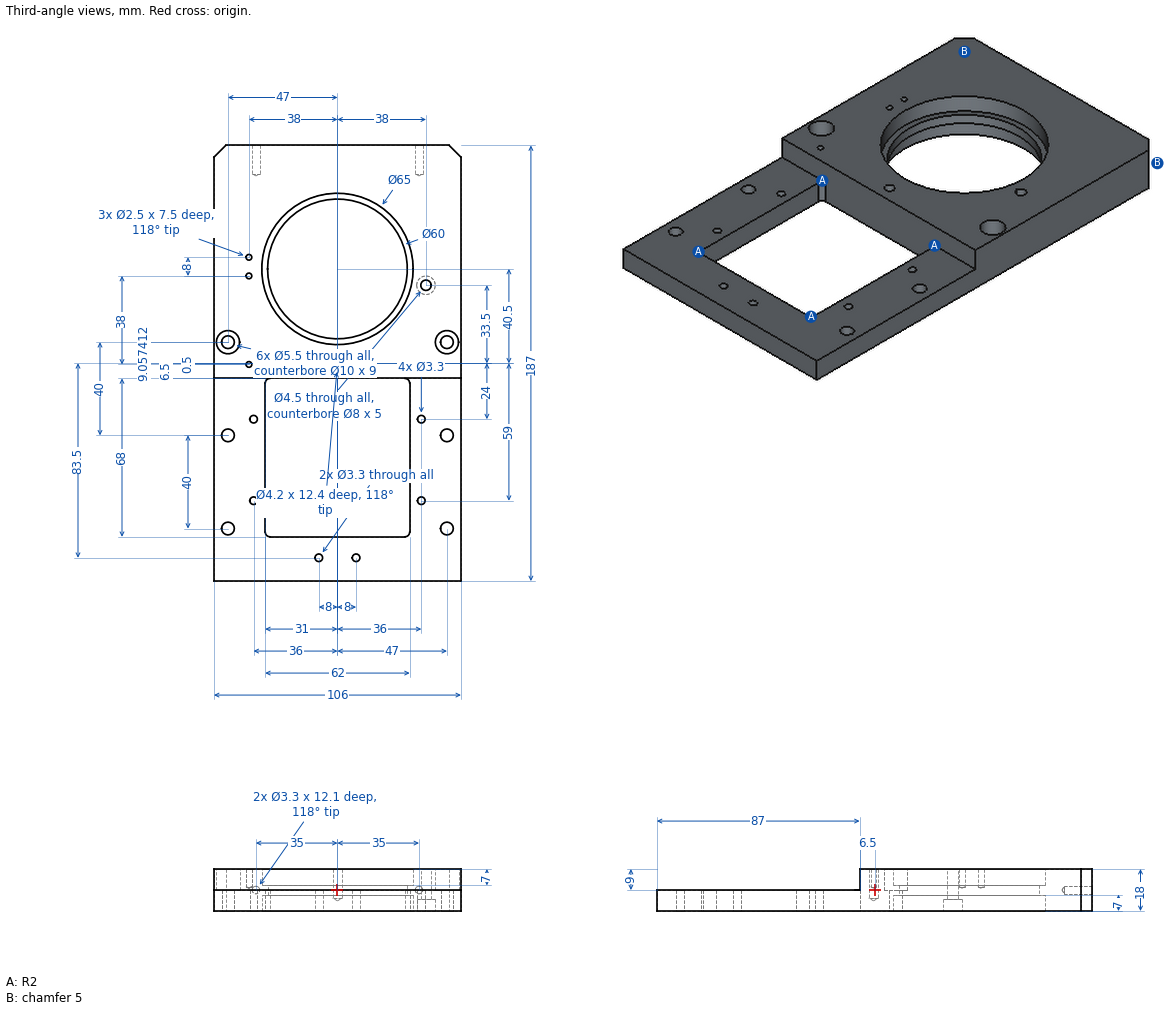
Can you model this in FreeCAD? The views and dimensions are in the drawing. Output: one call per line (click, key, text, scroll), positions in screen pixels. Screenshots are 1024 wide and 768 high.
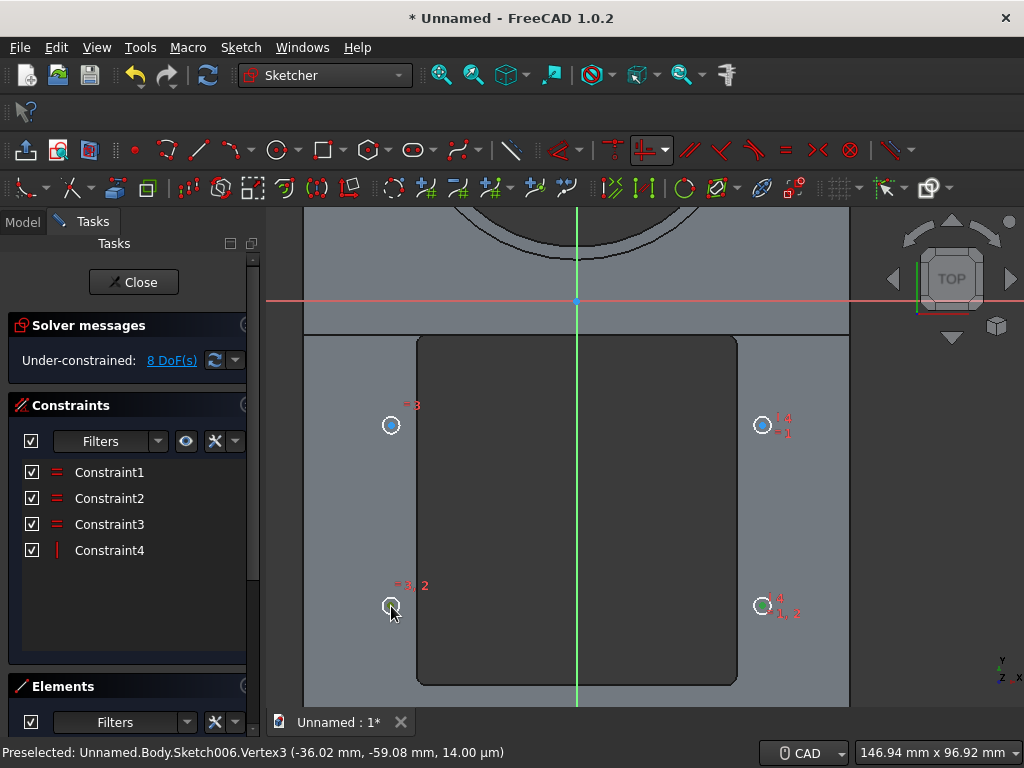
key(h)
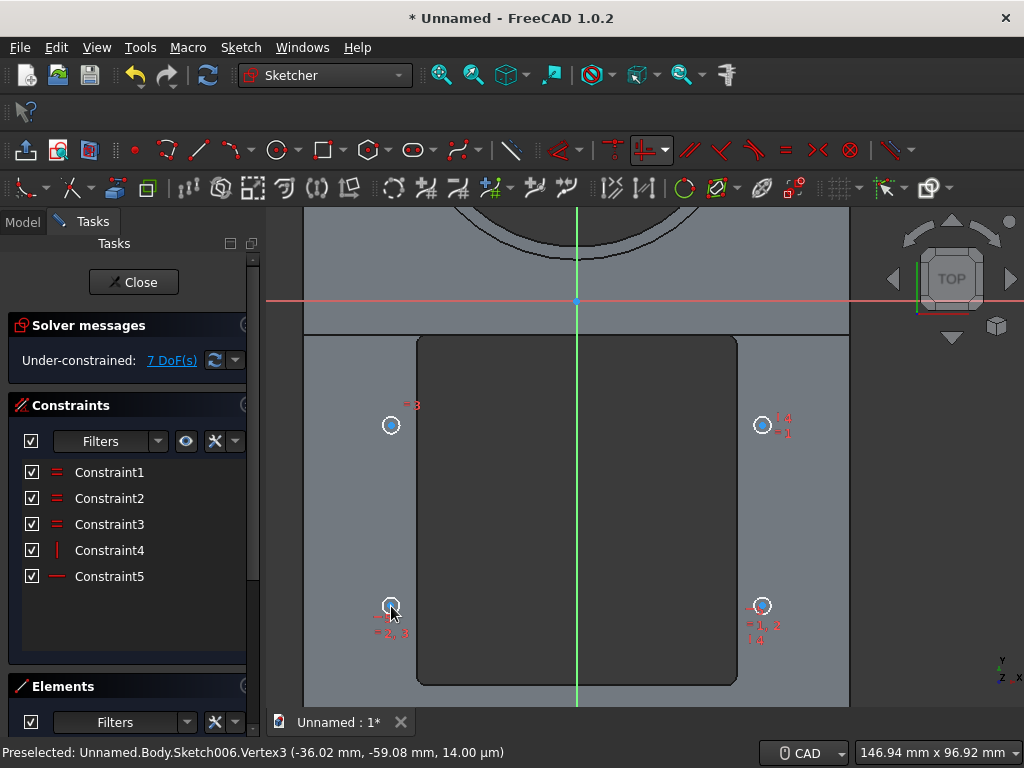
click(391, 606)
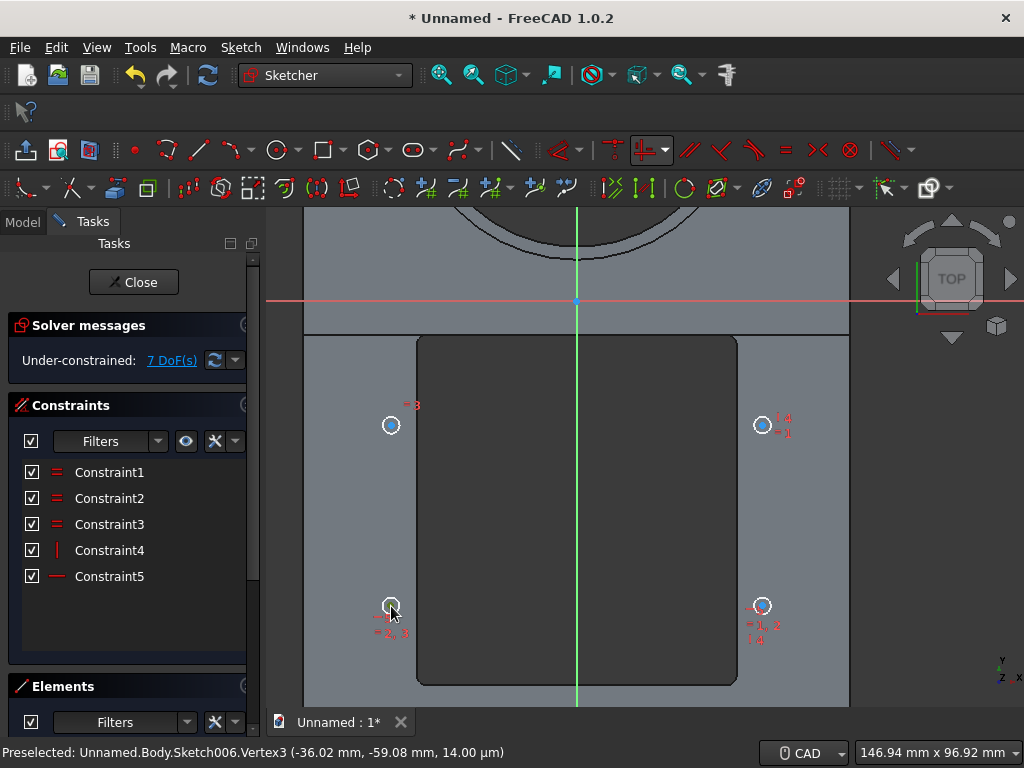
click(391, 425)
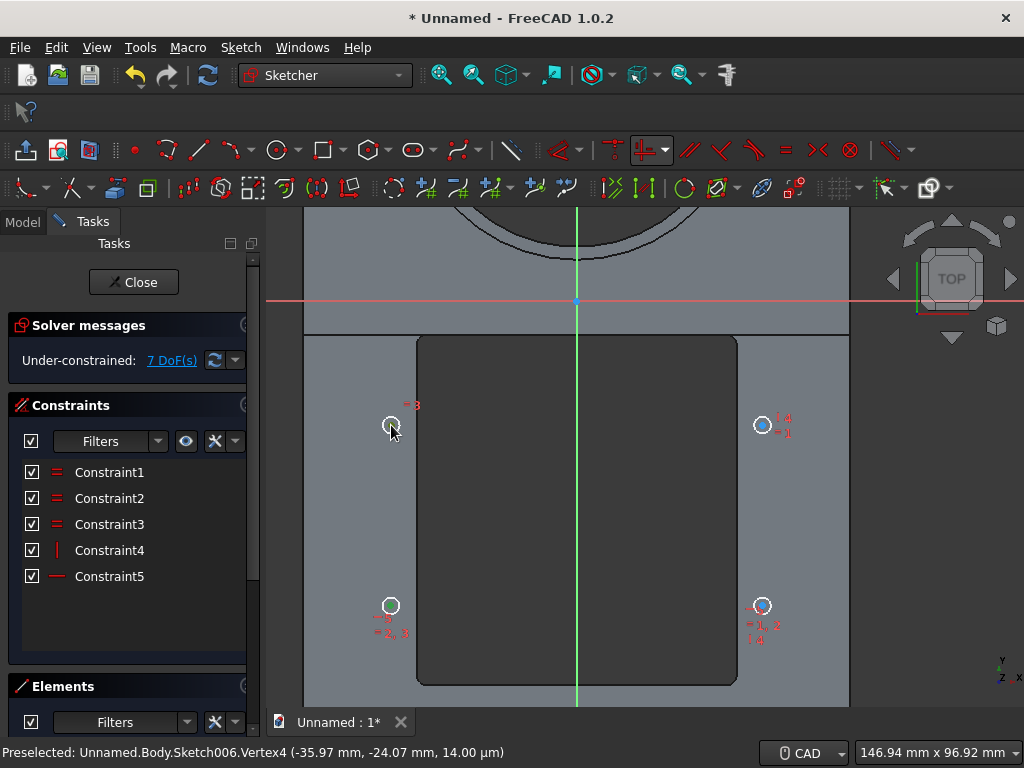
click(668, 150)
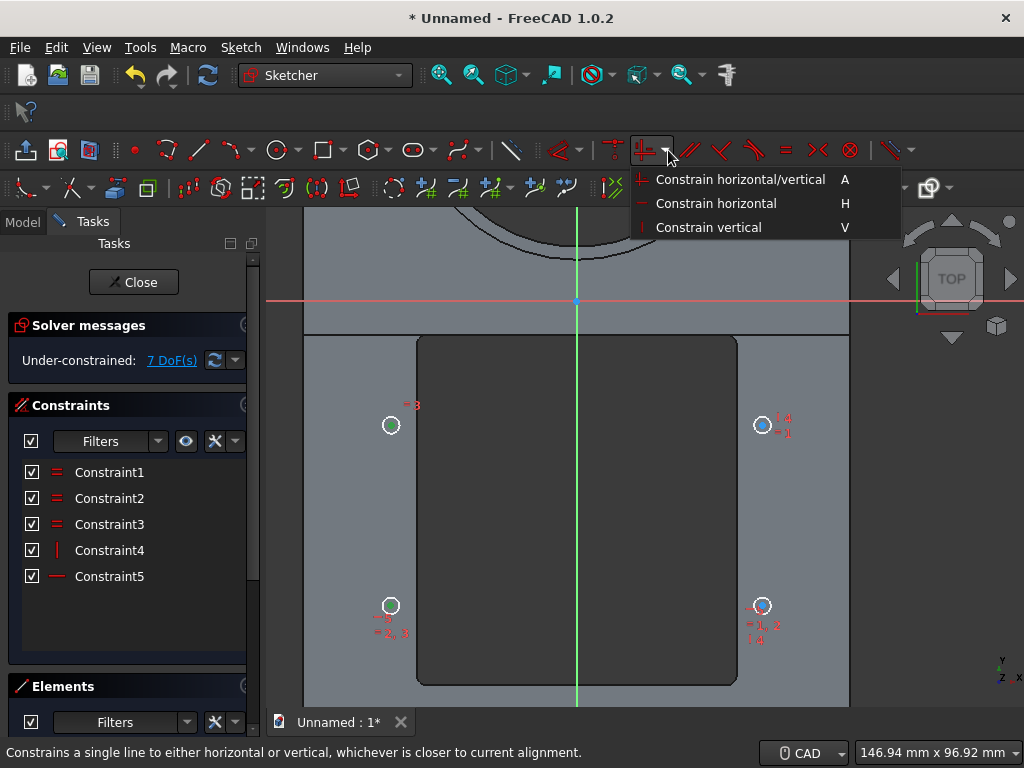
click(766, 227)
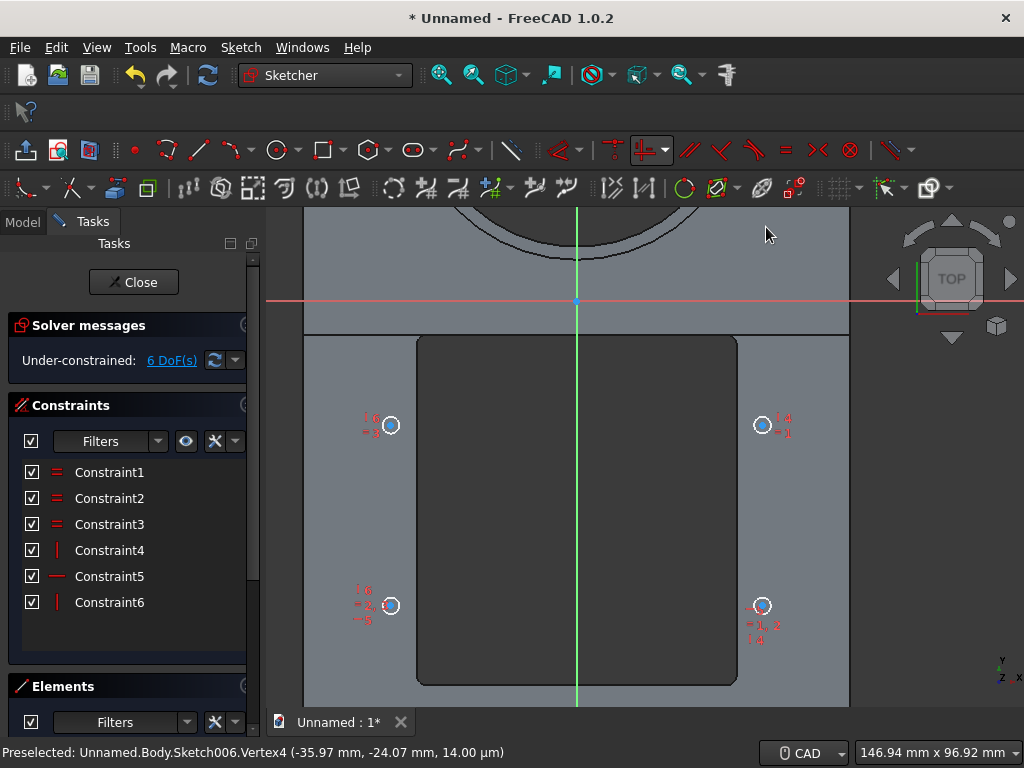
click(762, 425)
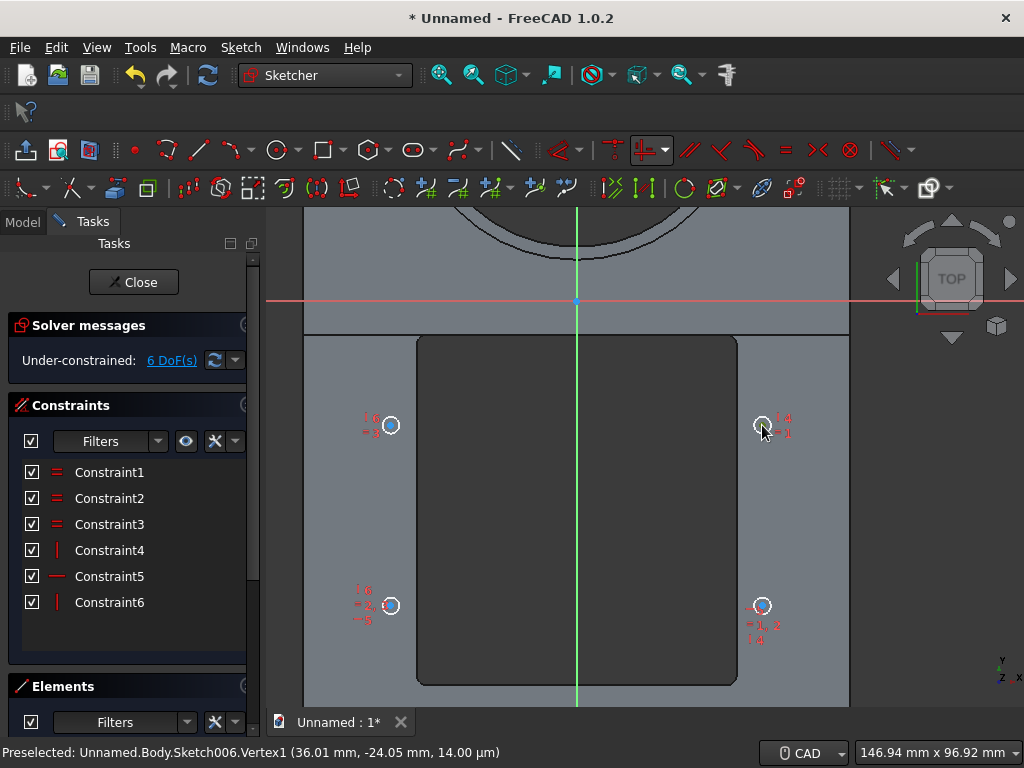
click(391, 425)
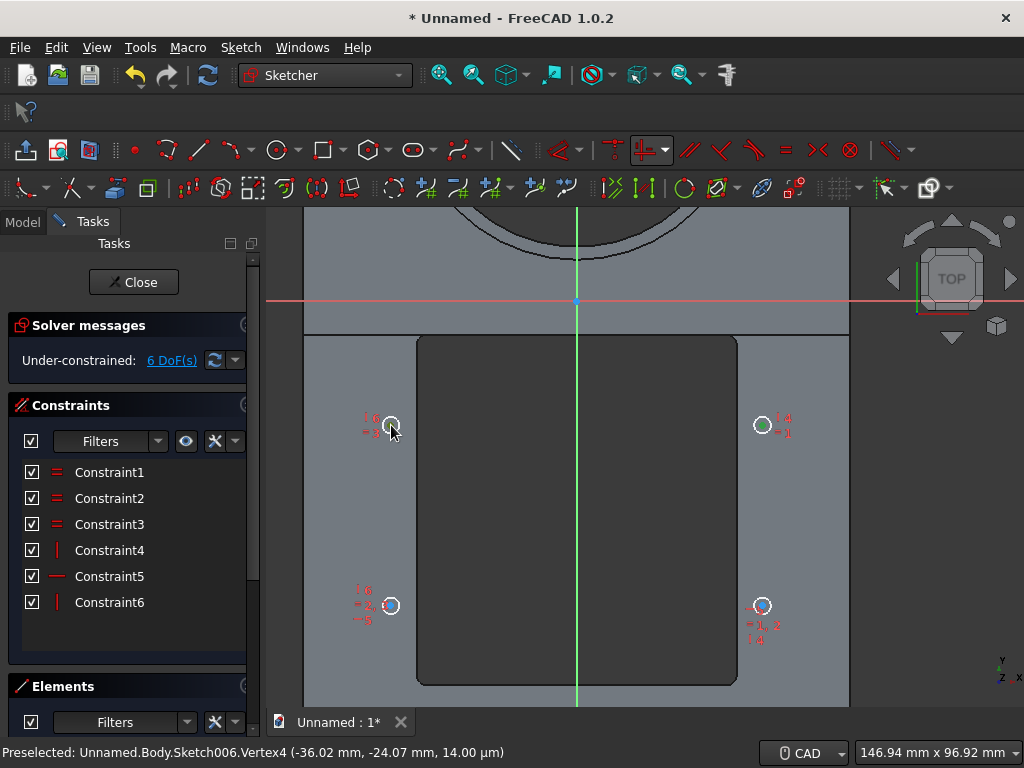
click(668, 150)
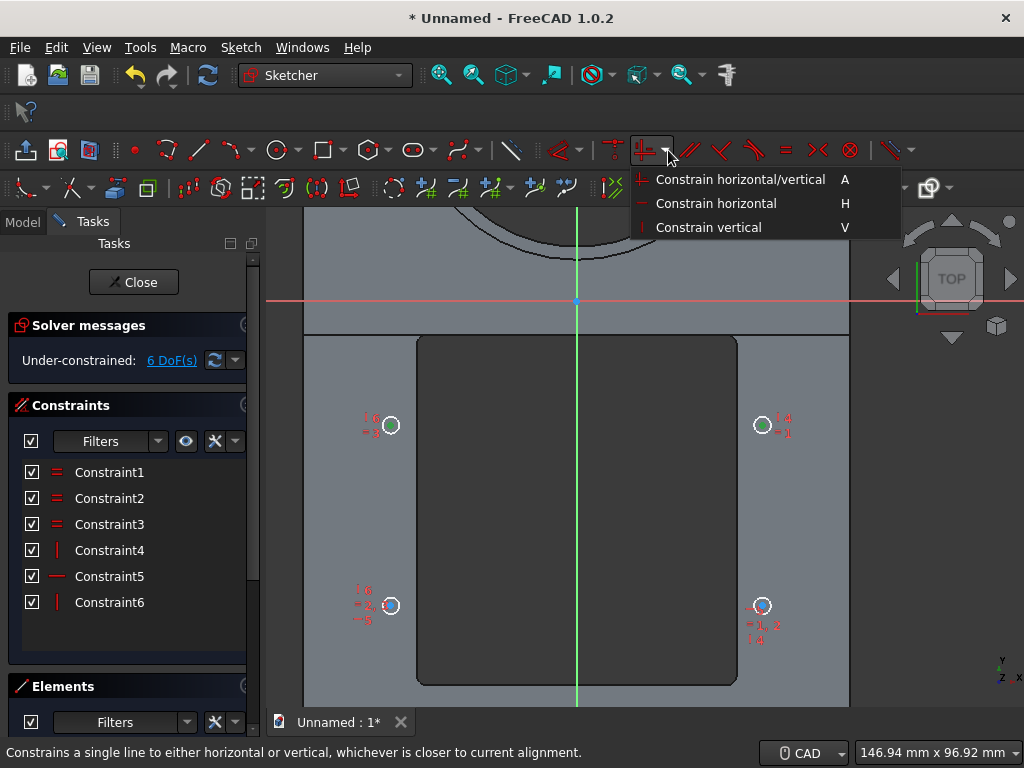
click(766, 203)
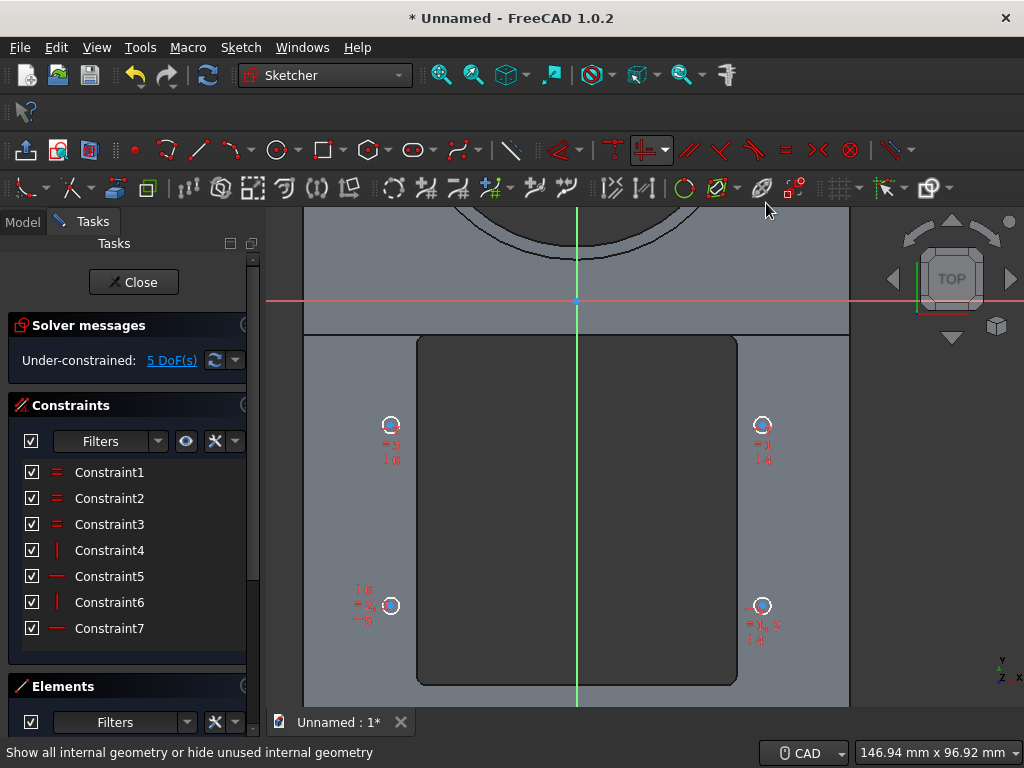
click(558, 150)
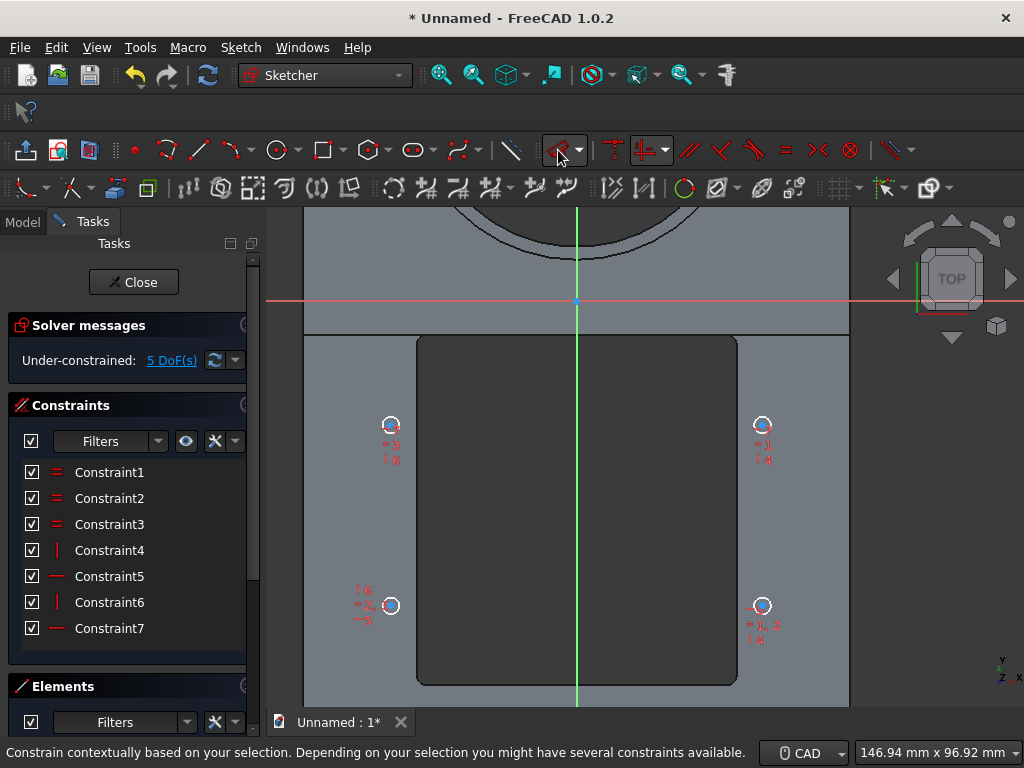
scroll(757, 431, up, 5)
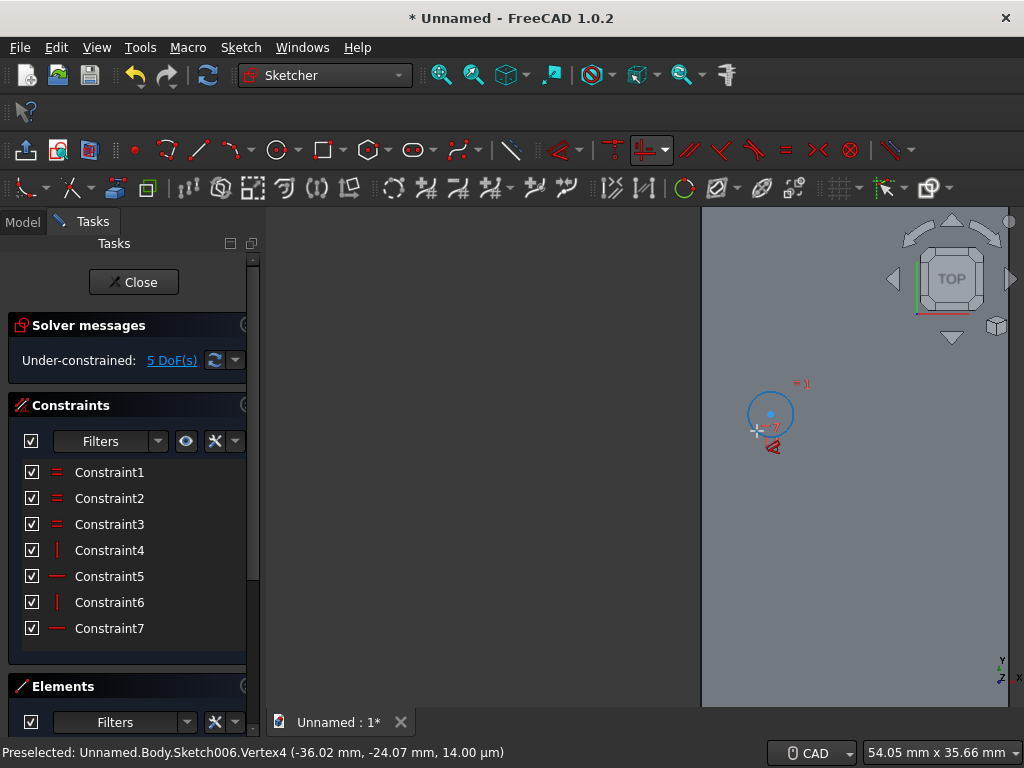
click(755, 430)
click(732, 452)